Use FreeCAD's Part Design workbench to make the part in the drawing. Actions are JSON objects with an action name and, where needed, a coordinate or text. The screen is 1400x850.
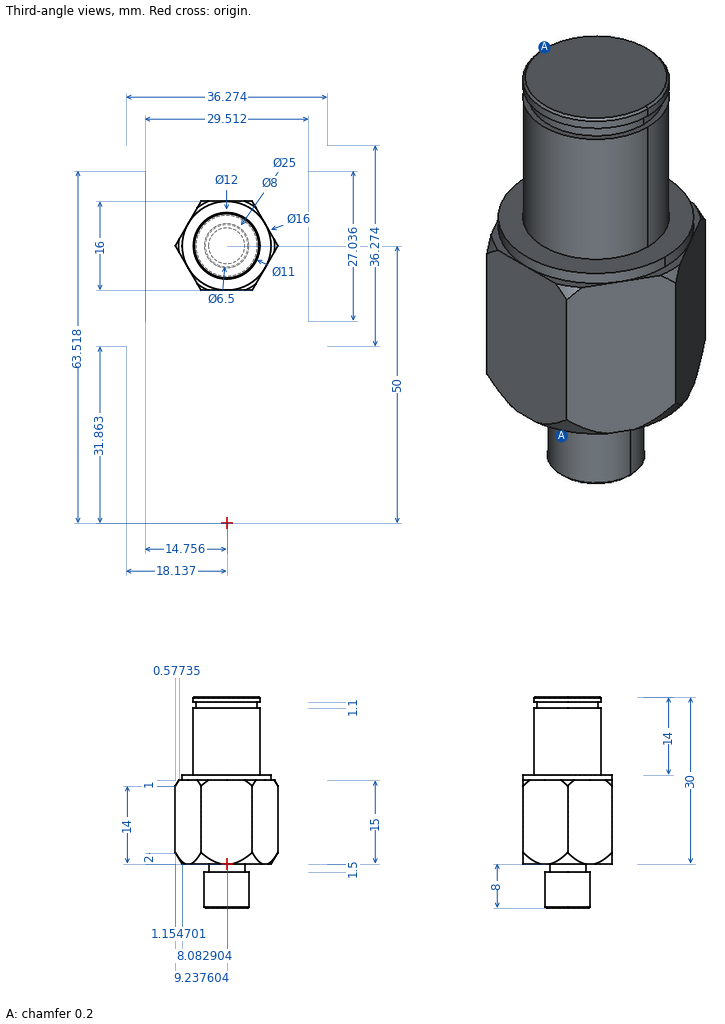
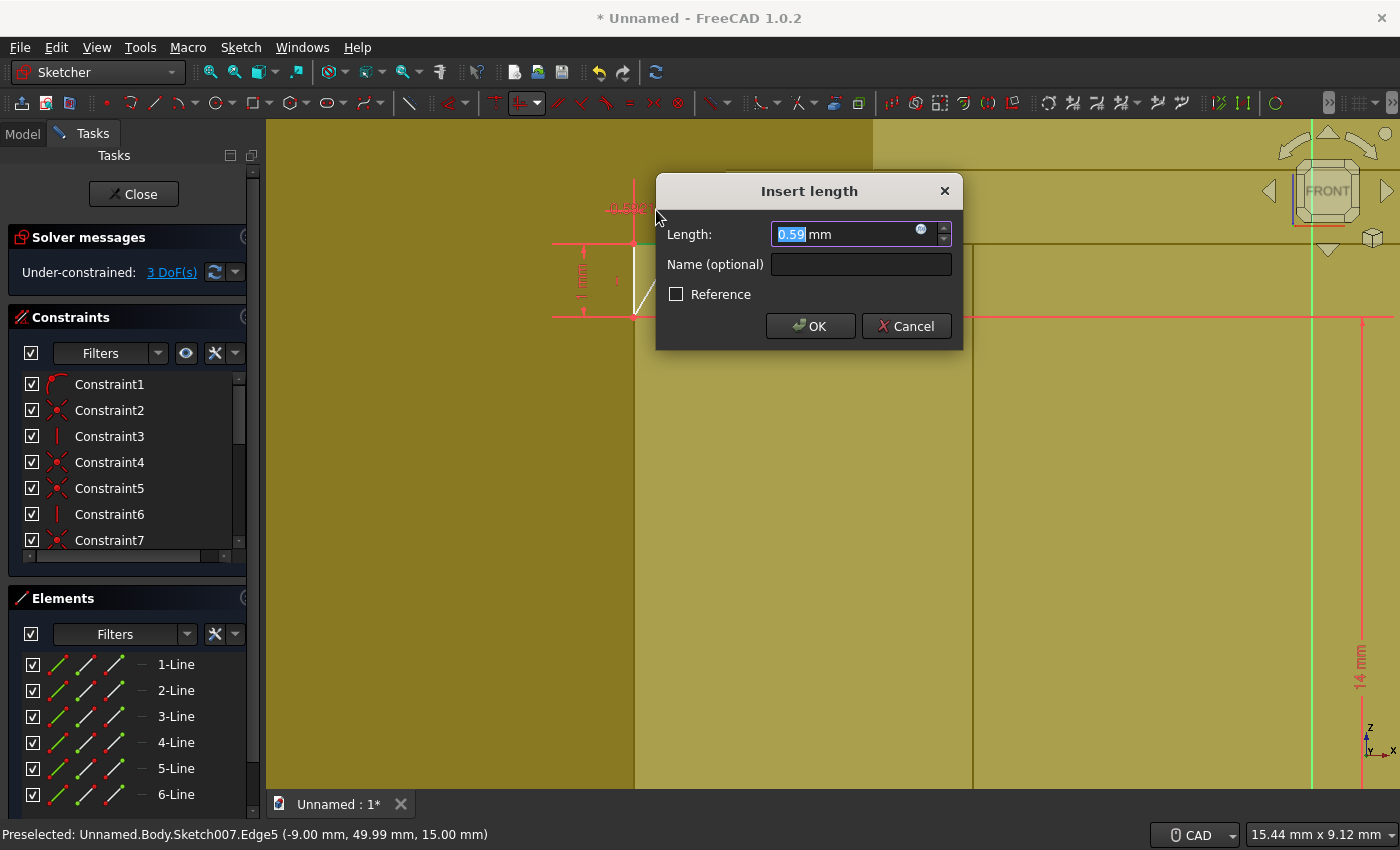
{"action": "type", "text": "0.57735"}
{"action": "key", "text": "Return"}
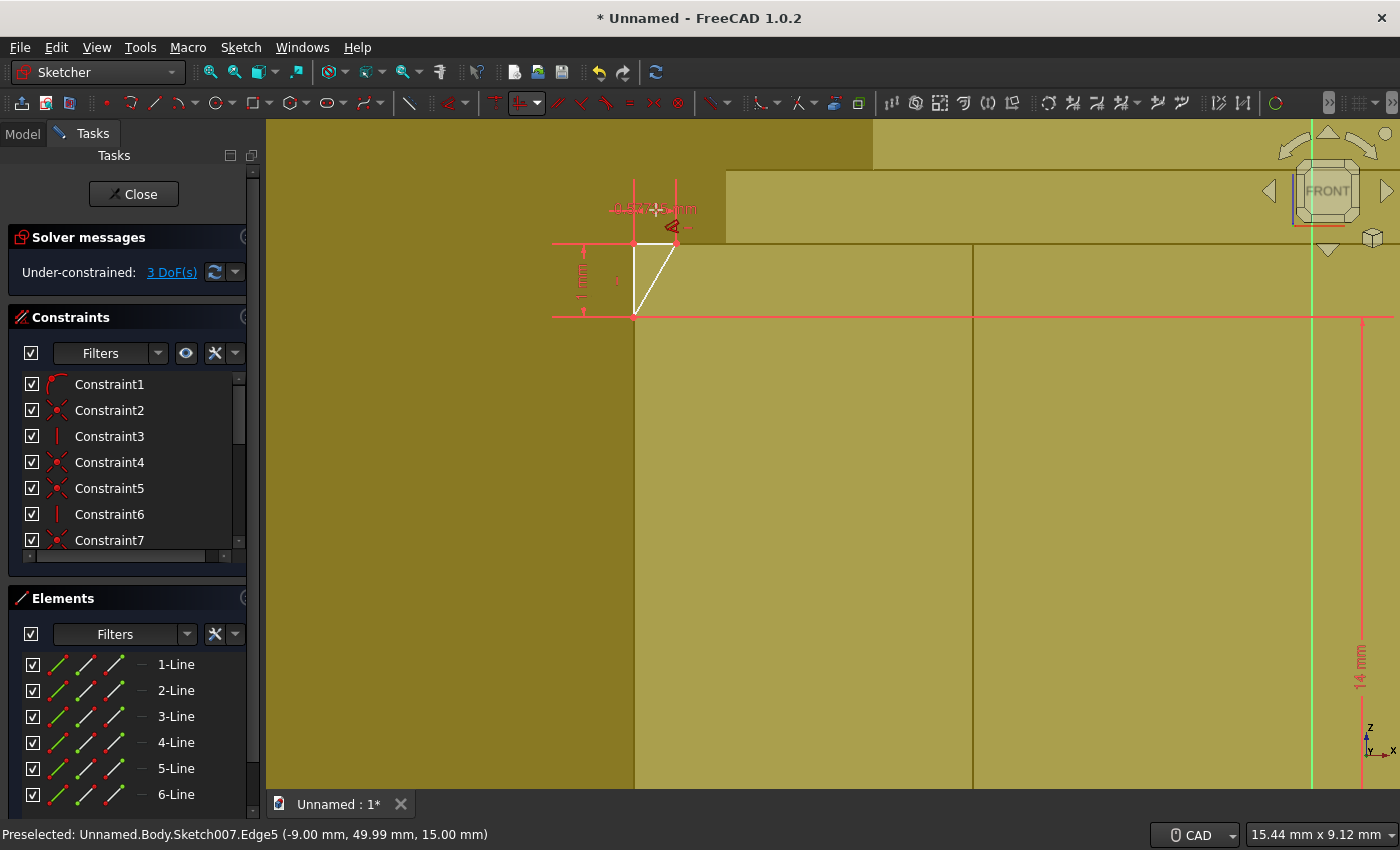
{"action": "scroll", "coordinate": [643, 256], "scroll_direction": "down", "scroll_amount": 5}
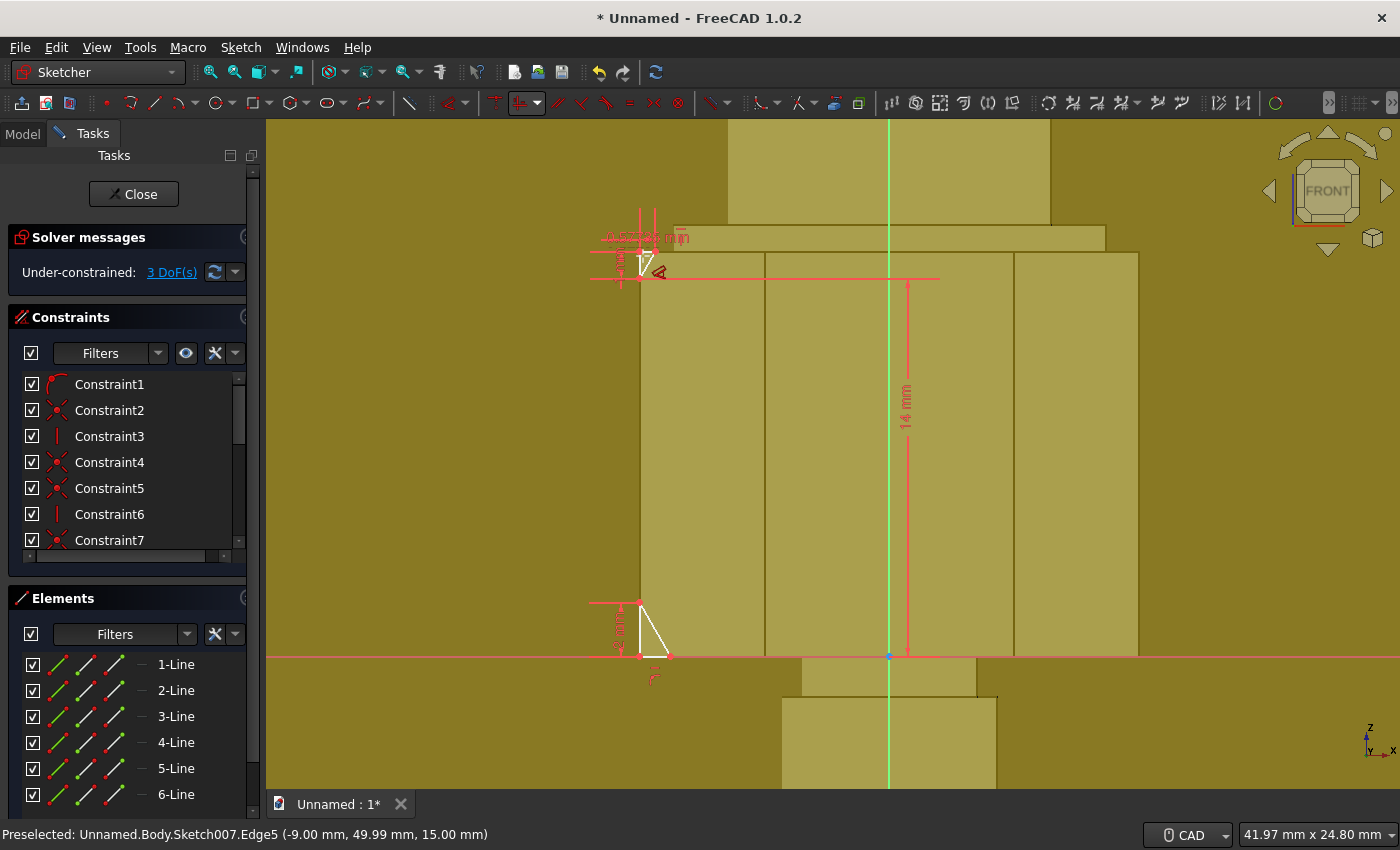
{"action": "scroll", "coordinate": [662, 657], "scroll_direction": "up", "scroll_amount": 3}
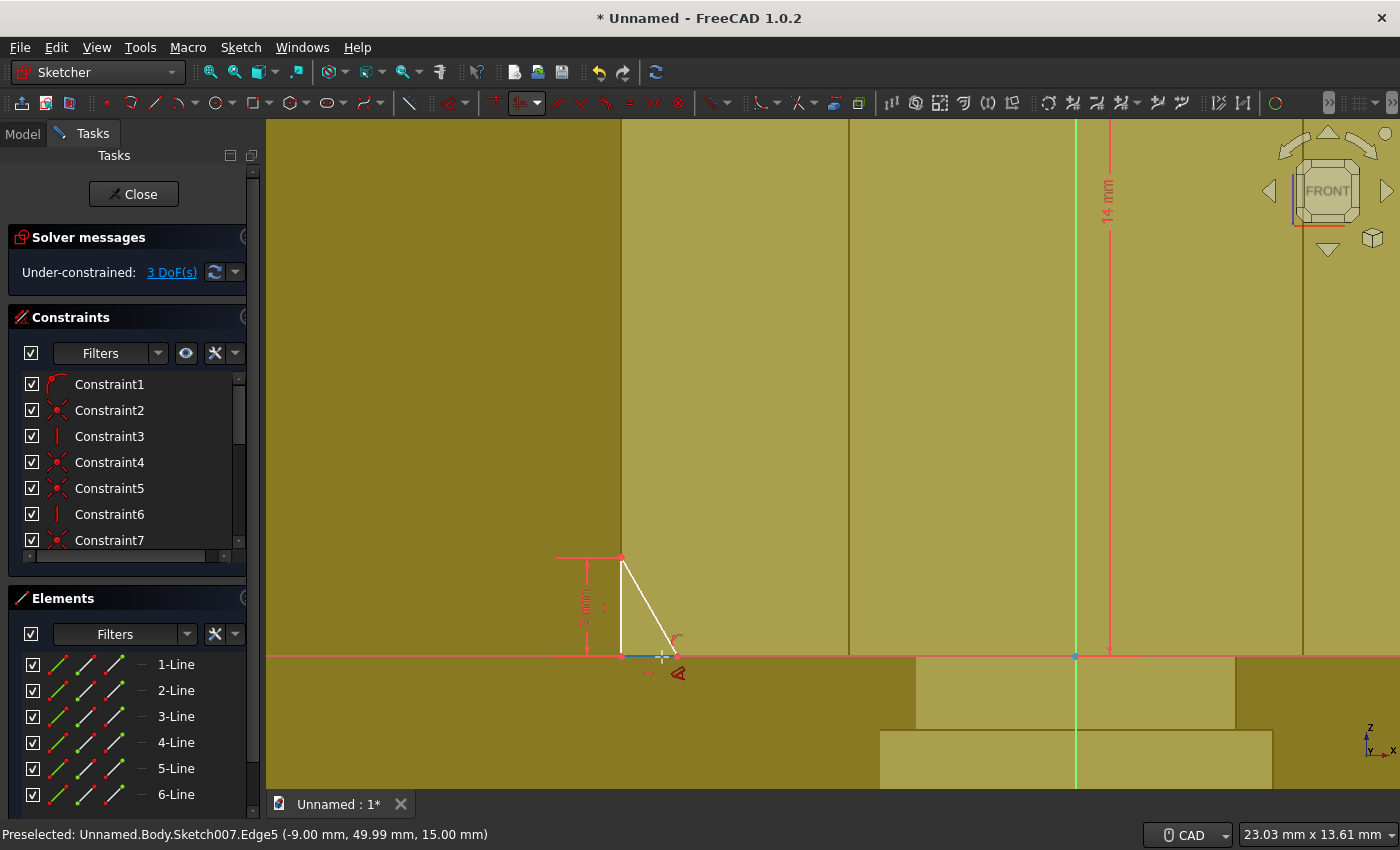
{"action": "left_click", "coordinate": [661, 656]}
{"action": "left_click", "coordinate": [650, 690]}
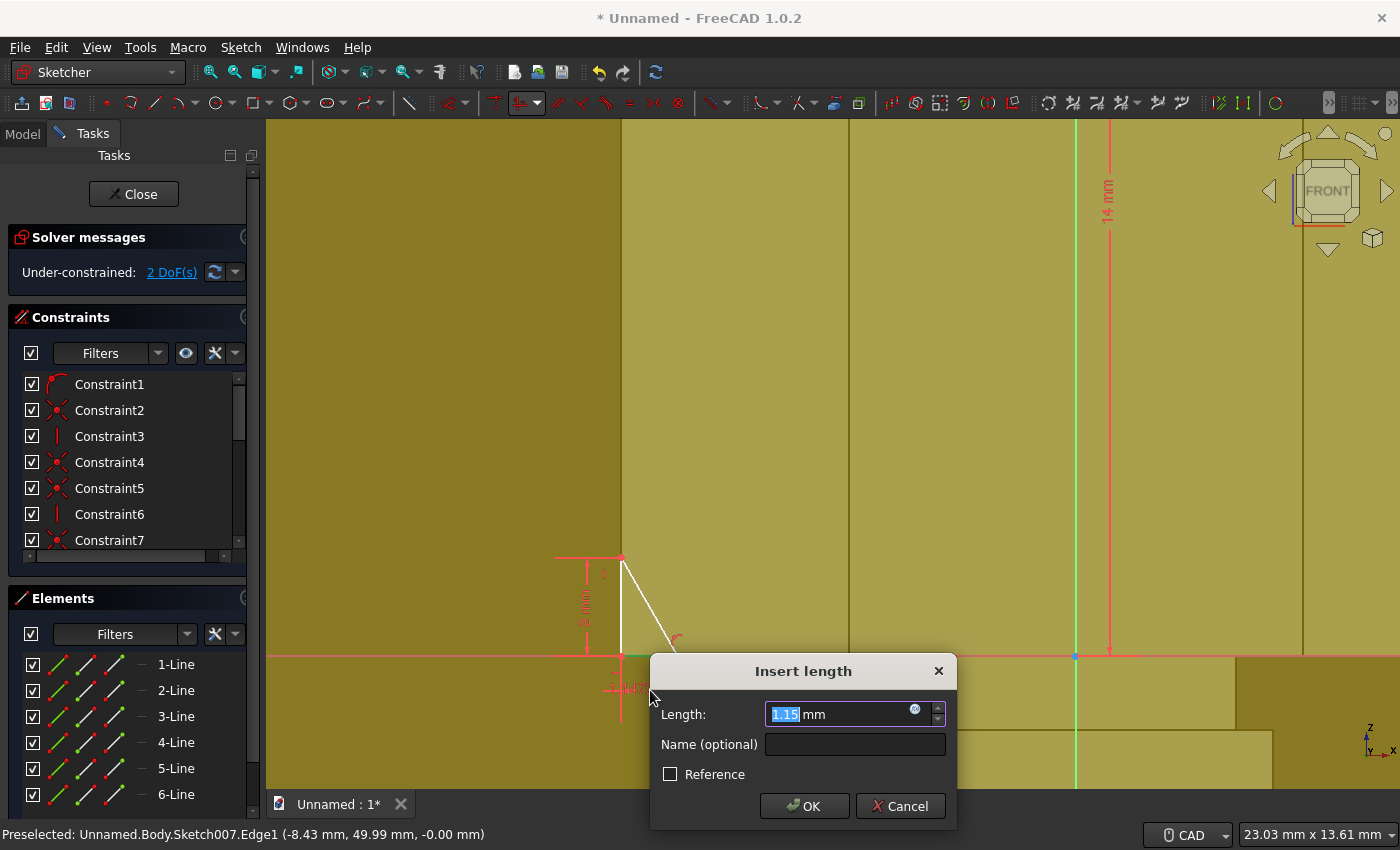
{"action": "type", "text": "1.154701"}
{"action": "key", "text": "Return"}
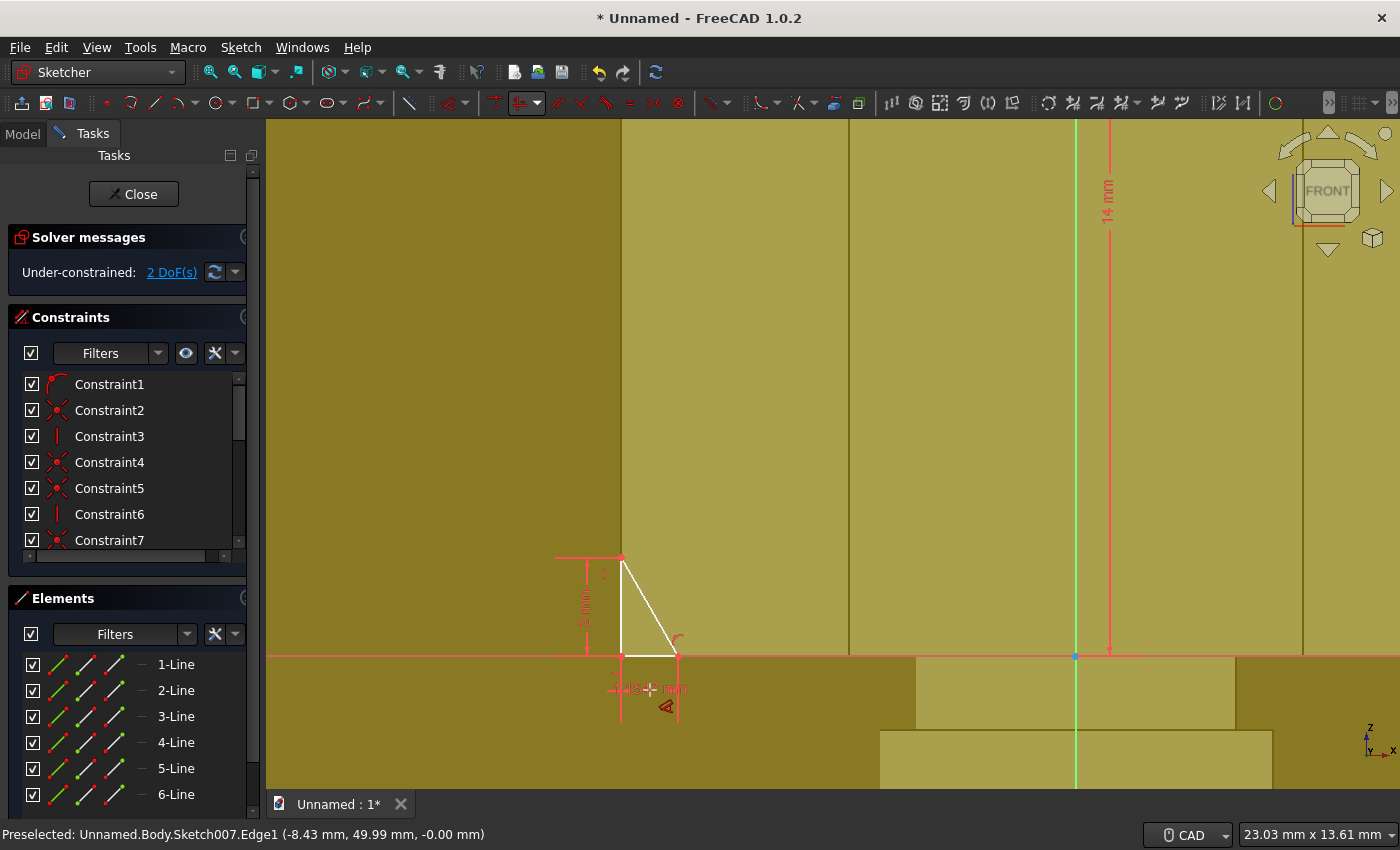
{"action": "left_click", "coordinate": [678, 656]}
{"action": "left_click", "coordinate": [877, 690]}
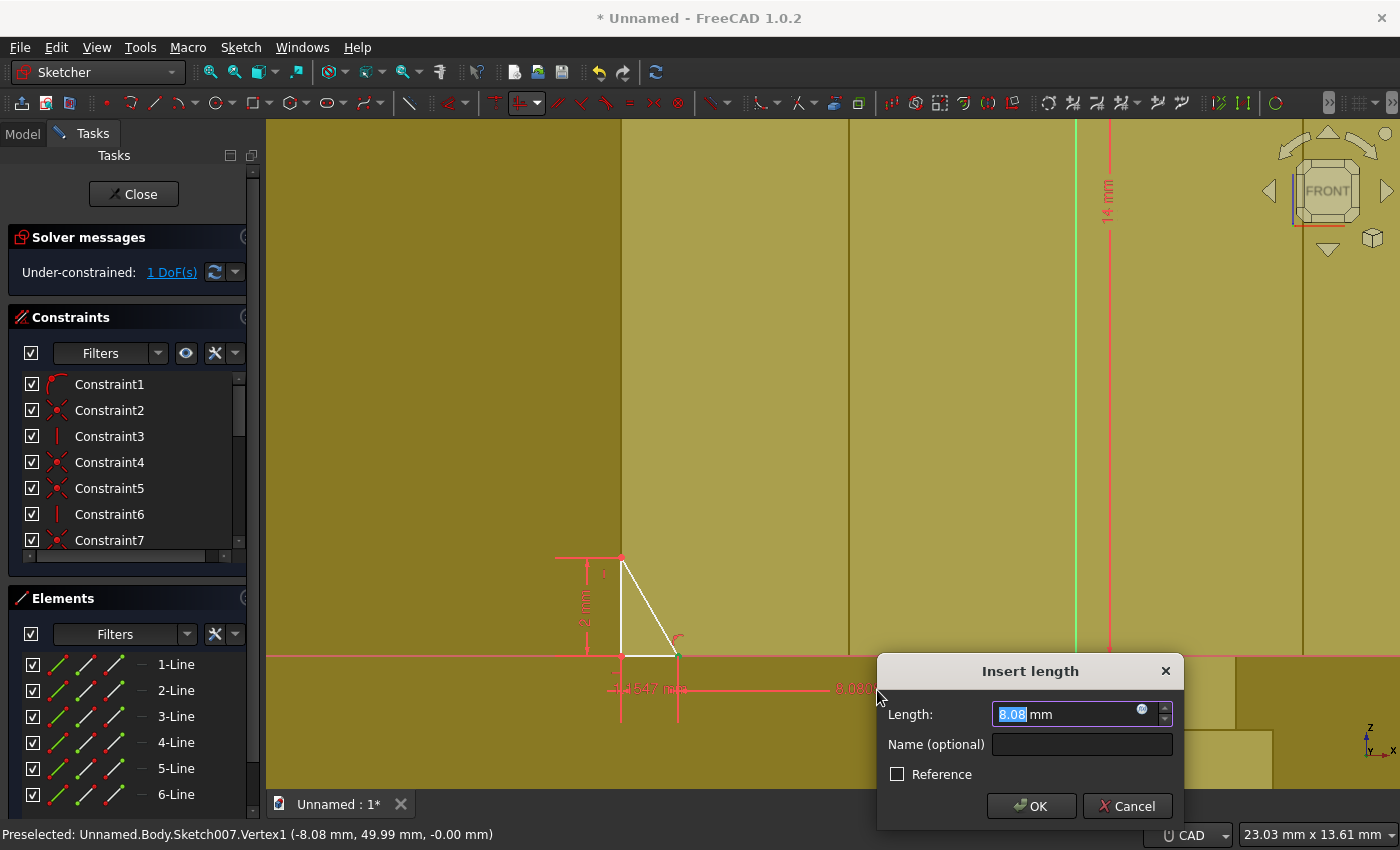
{"action": "type", "text": "8.082904"}
{"action": "key", "text": "Return"}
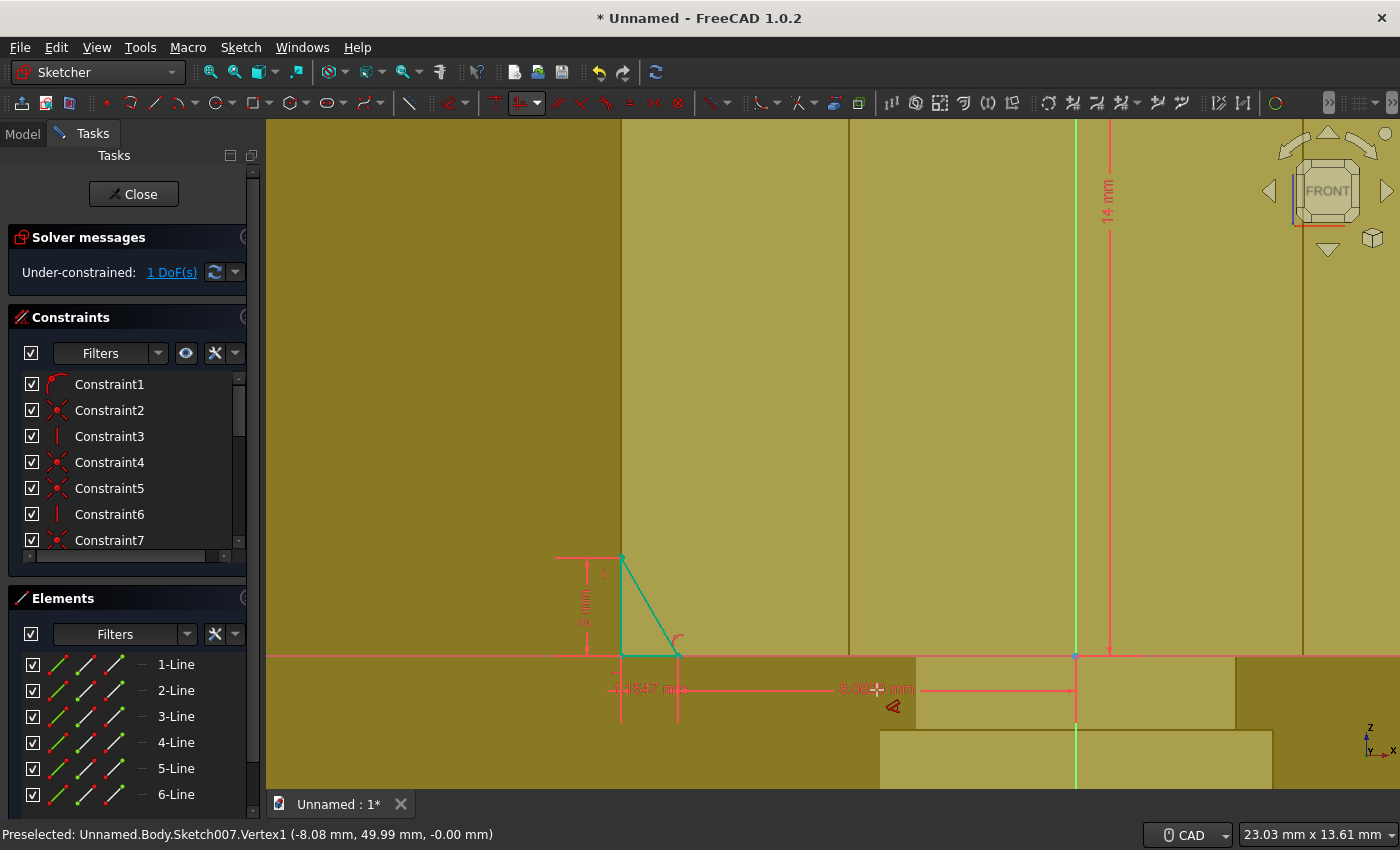
{"action": "scroll", "coordinate": [662, 657], "scroll_direction": "down", "scroll_amount": 3}